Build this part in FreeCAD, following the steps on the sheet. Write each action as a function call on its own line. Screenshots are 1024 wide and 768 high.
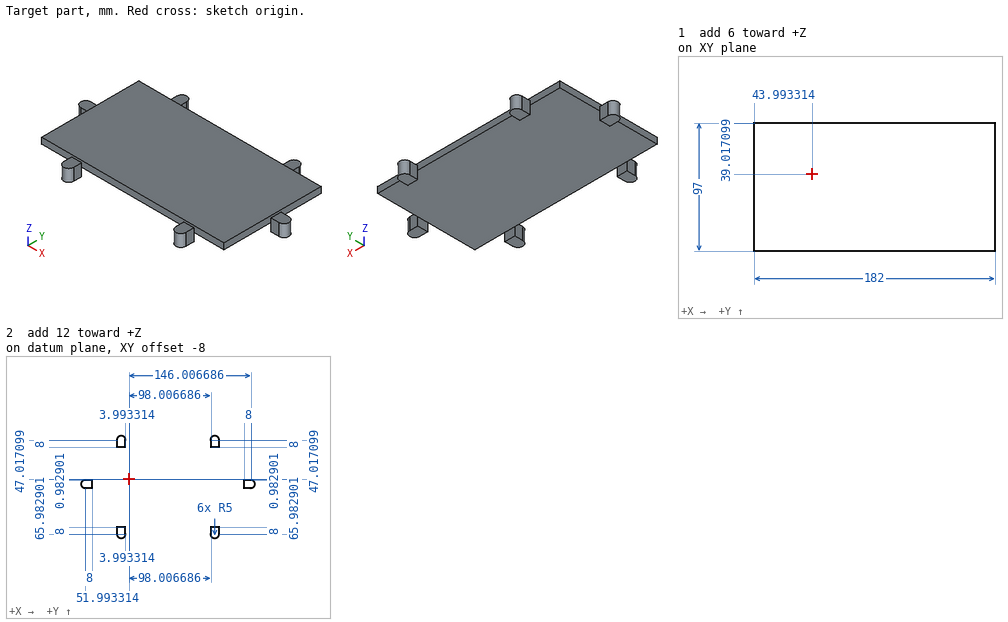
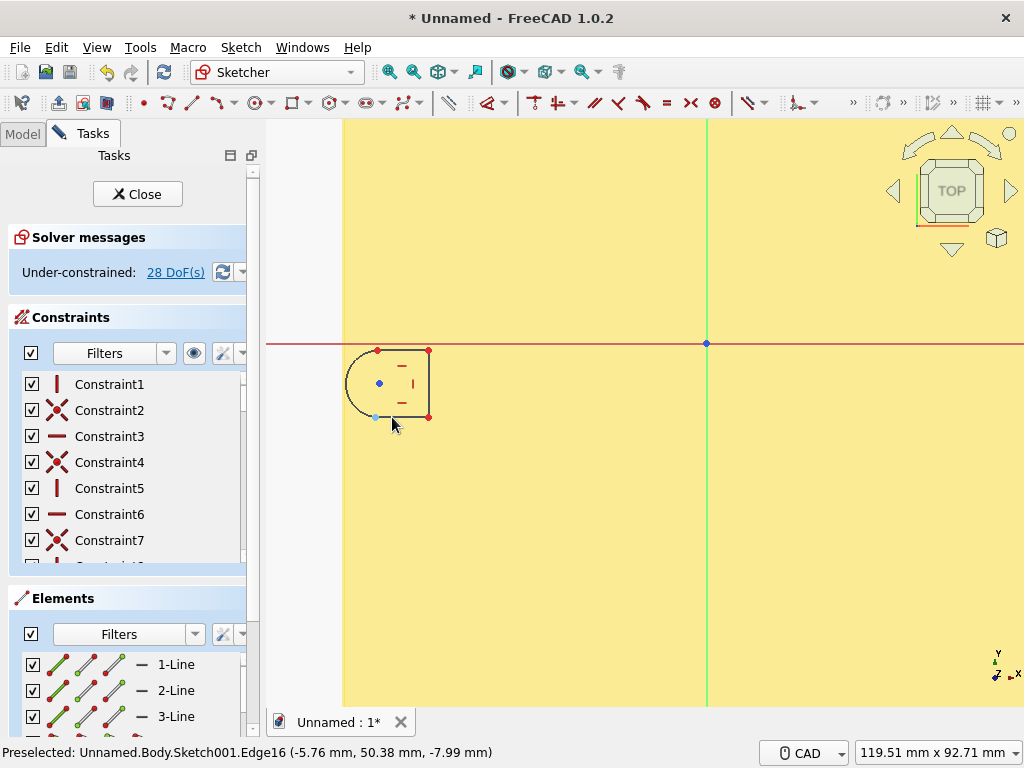
click(391, 417)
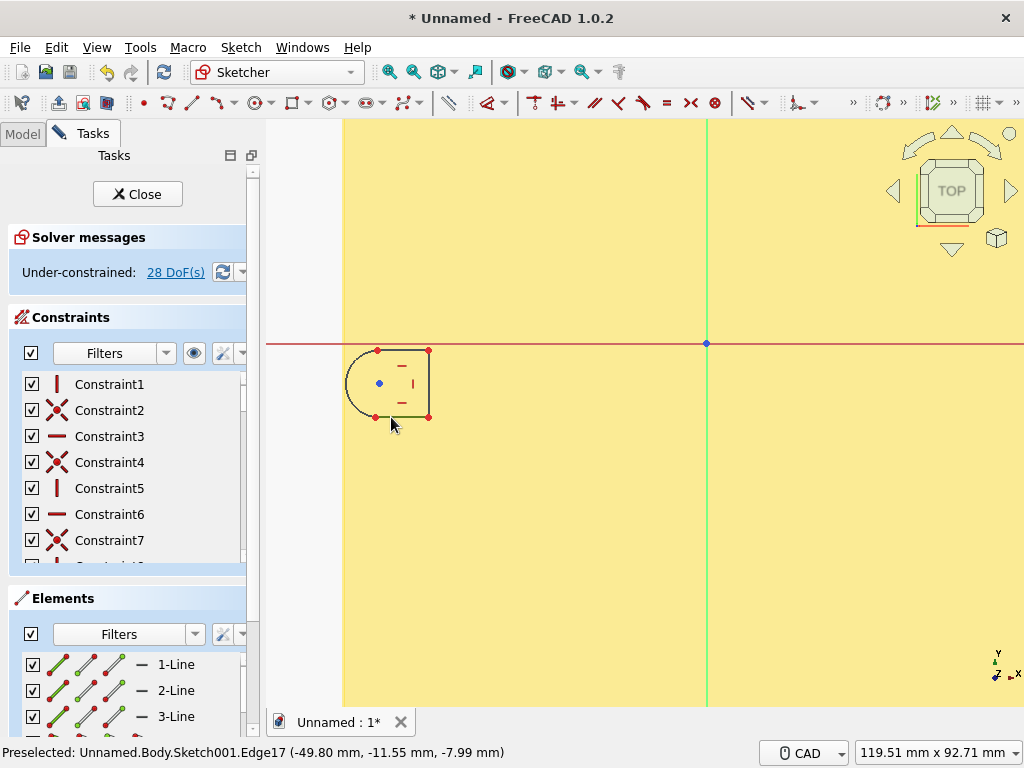
click(352, 365)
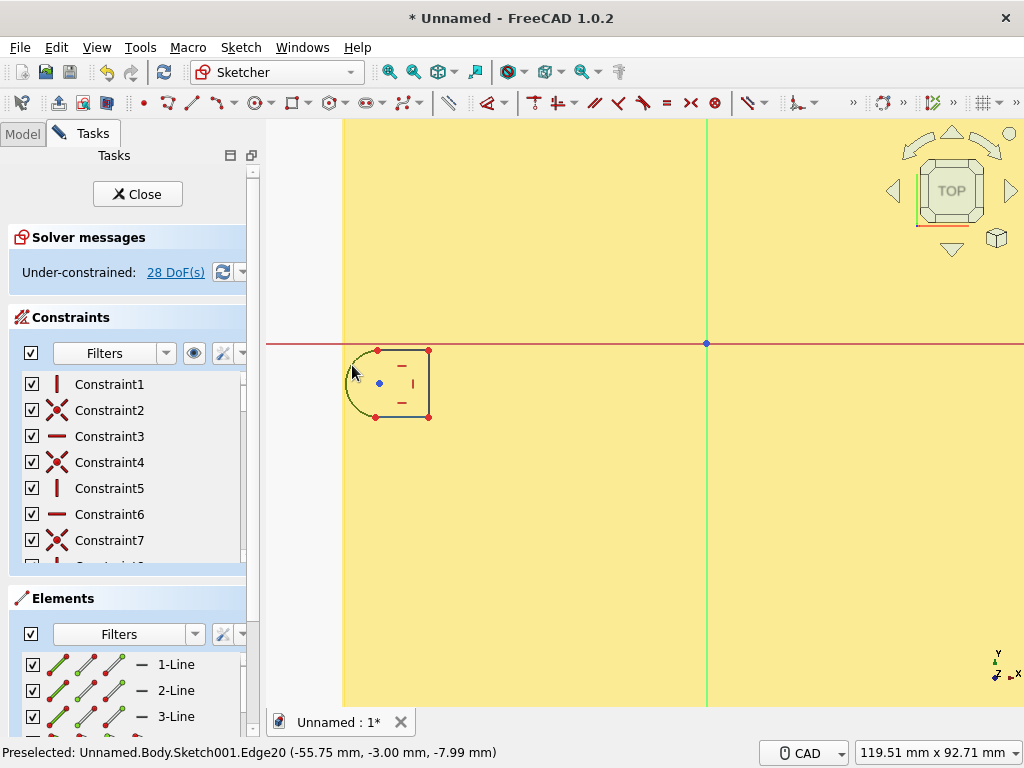
click(644, 104)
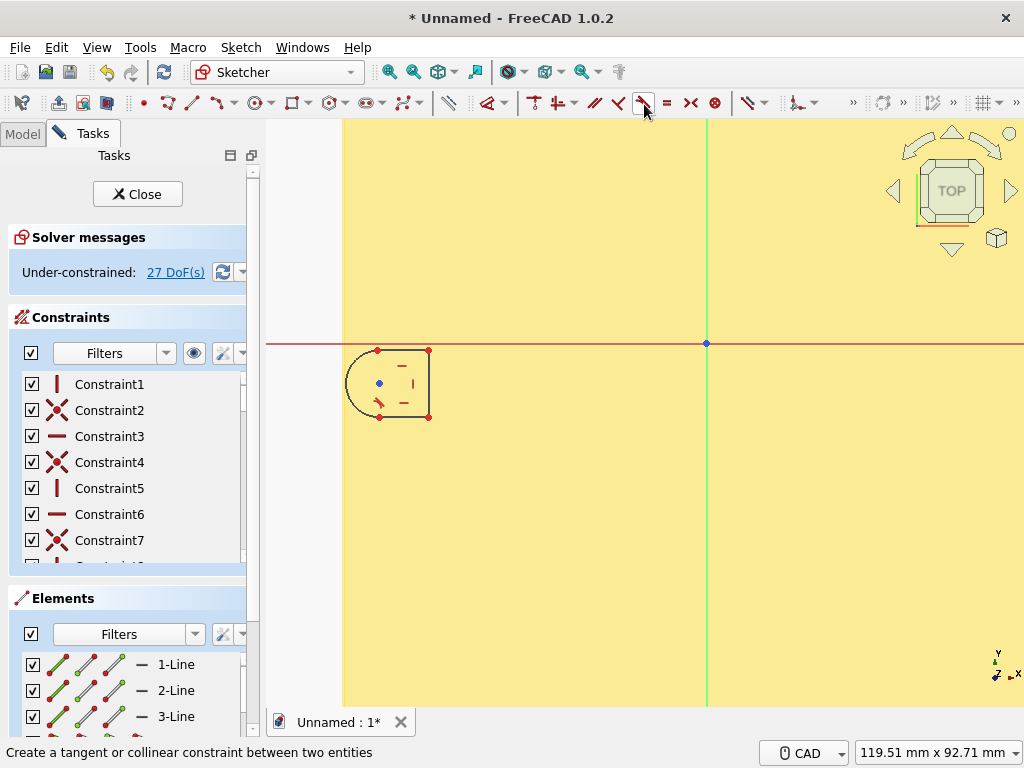
scroll(413, 350, up, 4)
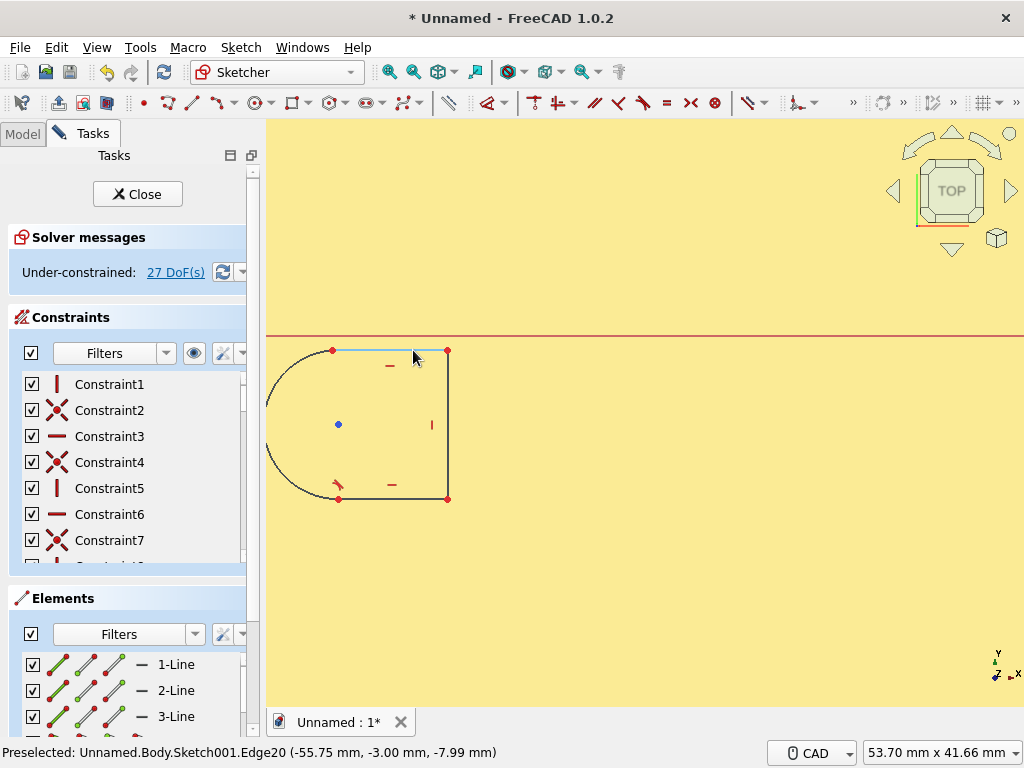
click(413, 350)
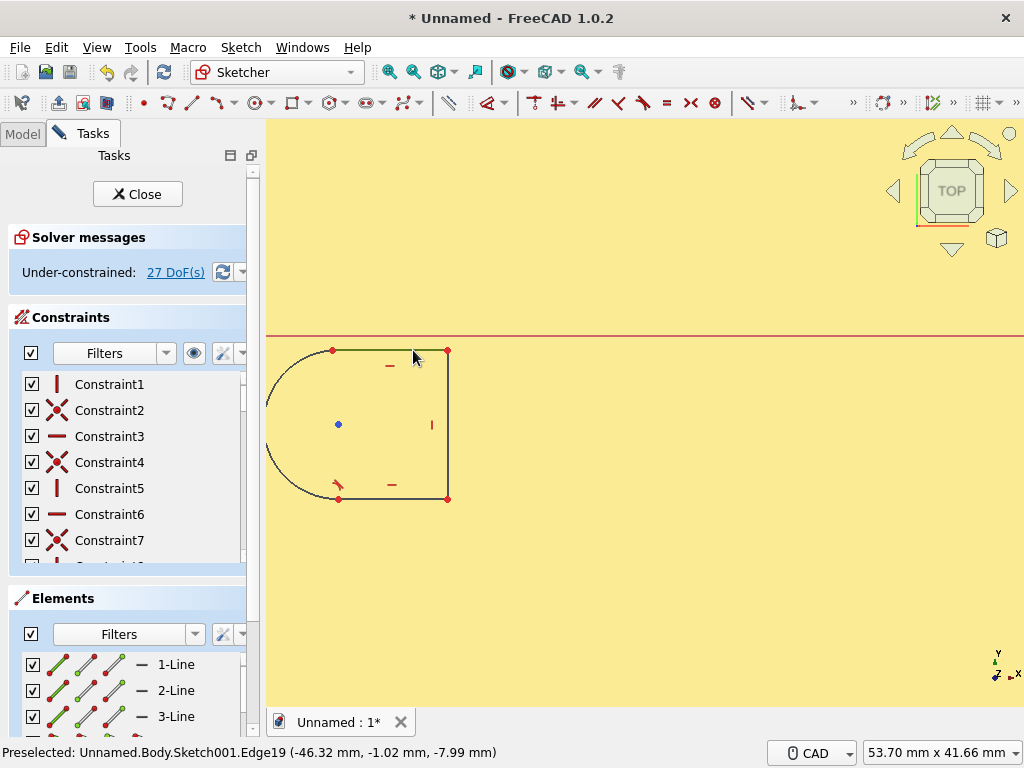
scroll(396, 404, down, 10)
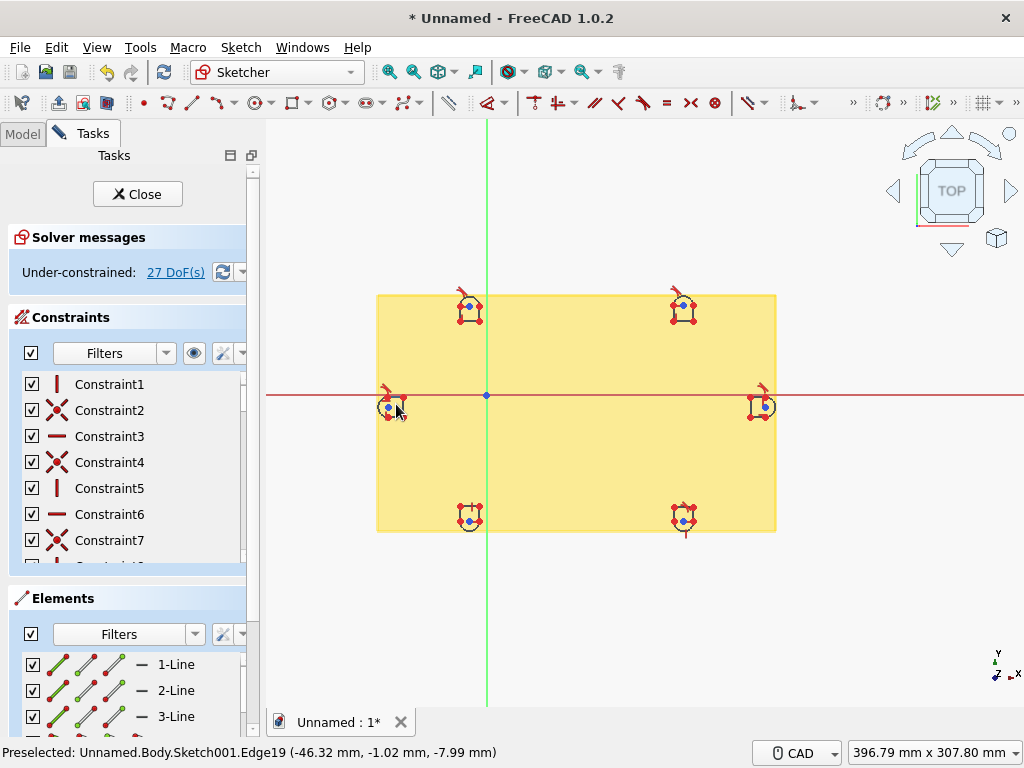
scroll(383, 415, up, 5)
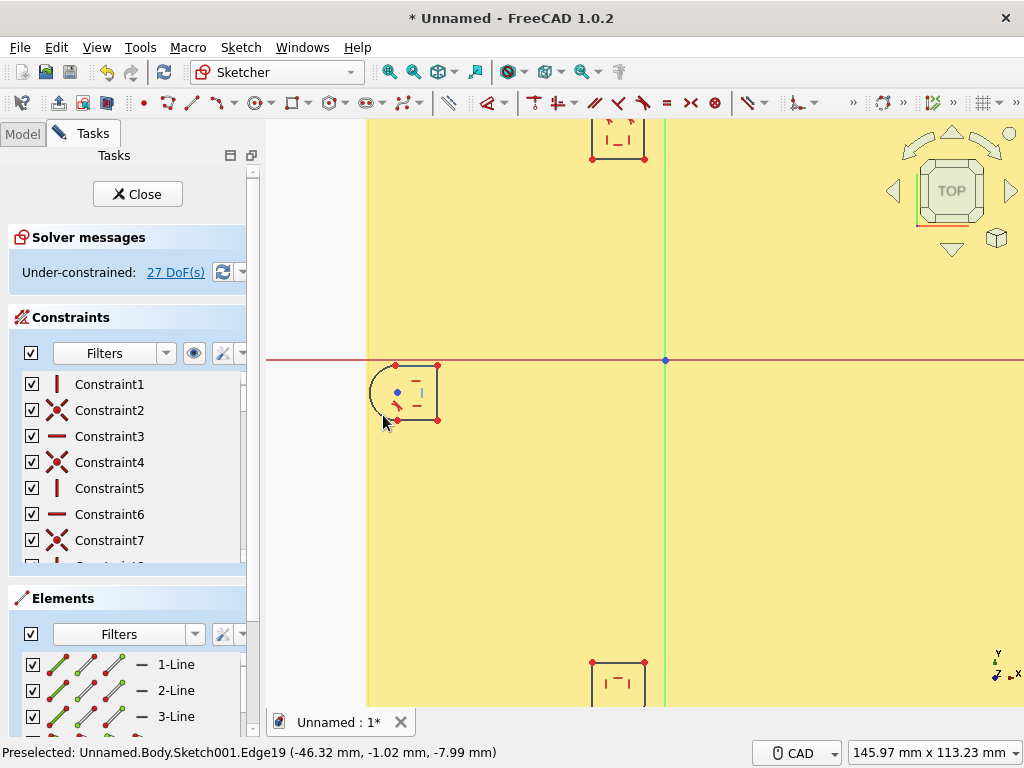
click(381, 415)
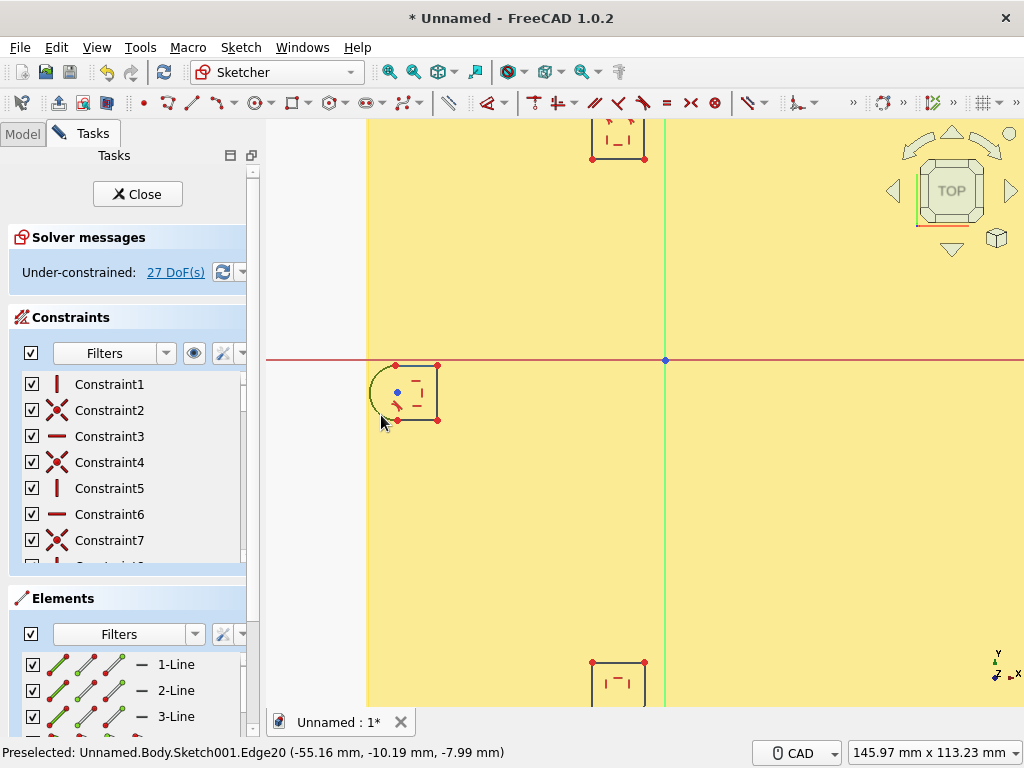
click(644, 104)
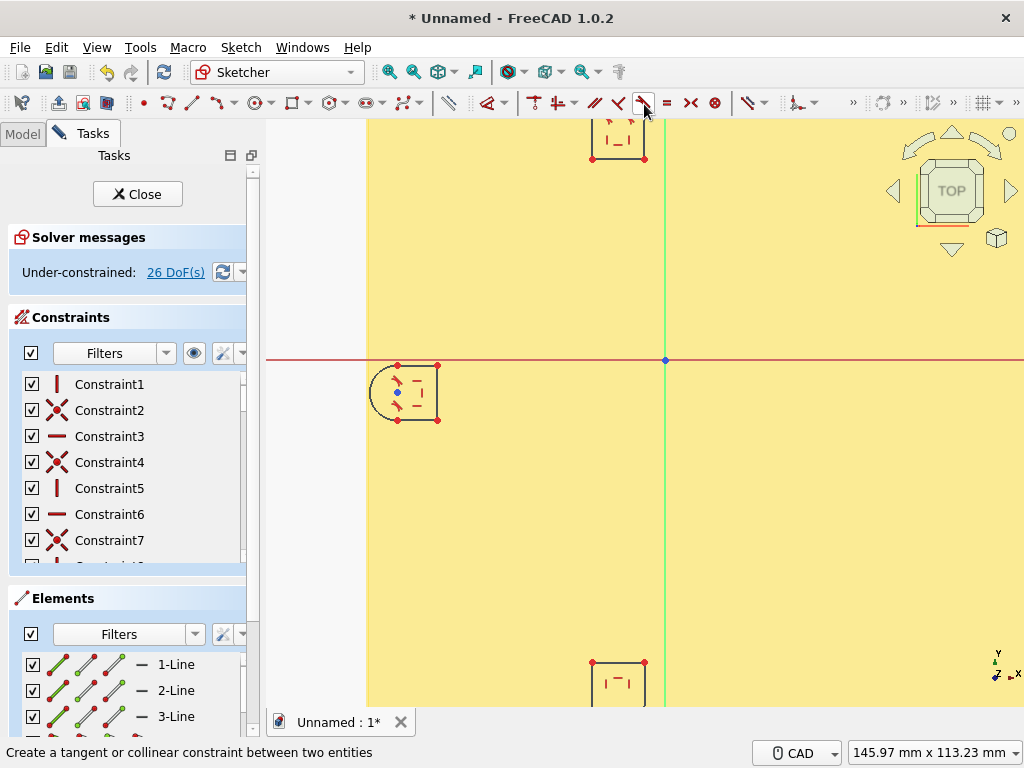
click(645, 675)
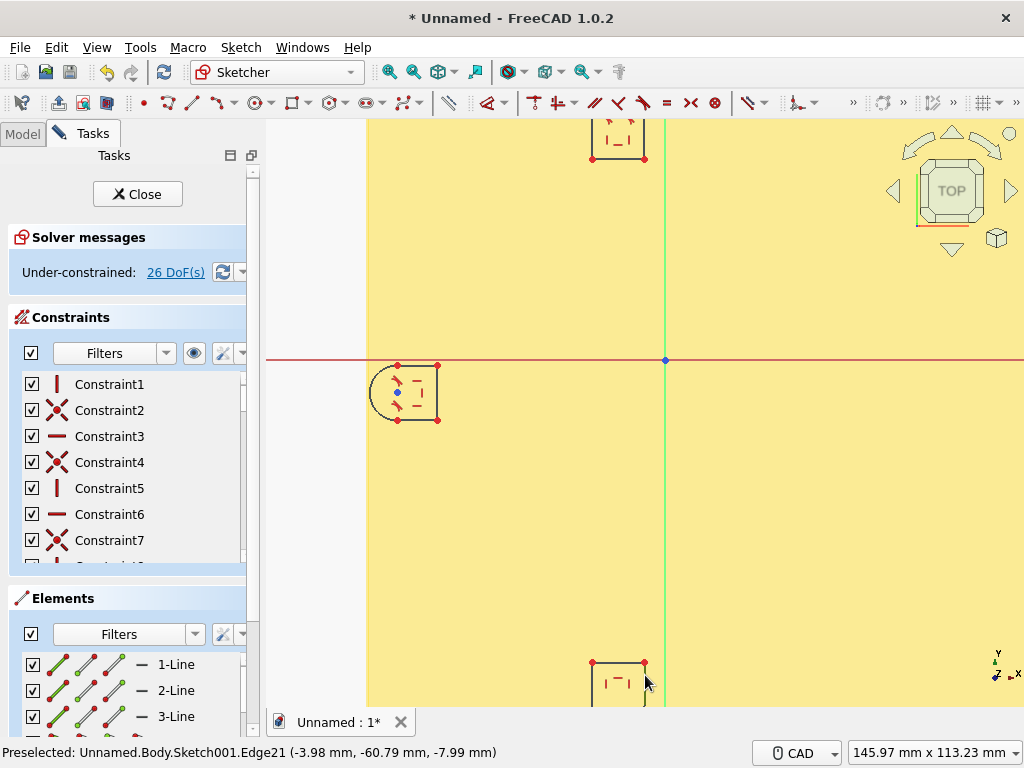
scroll(383, 415, down, 5)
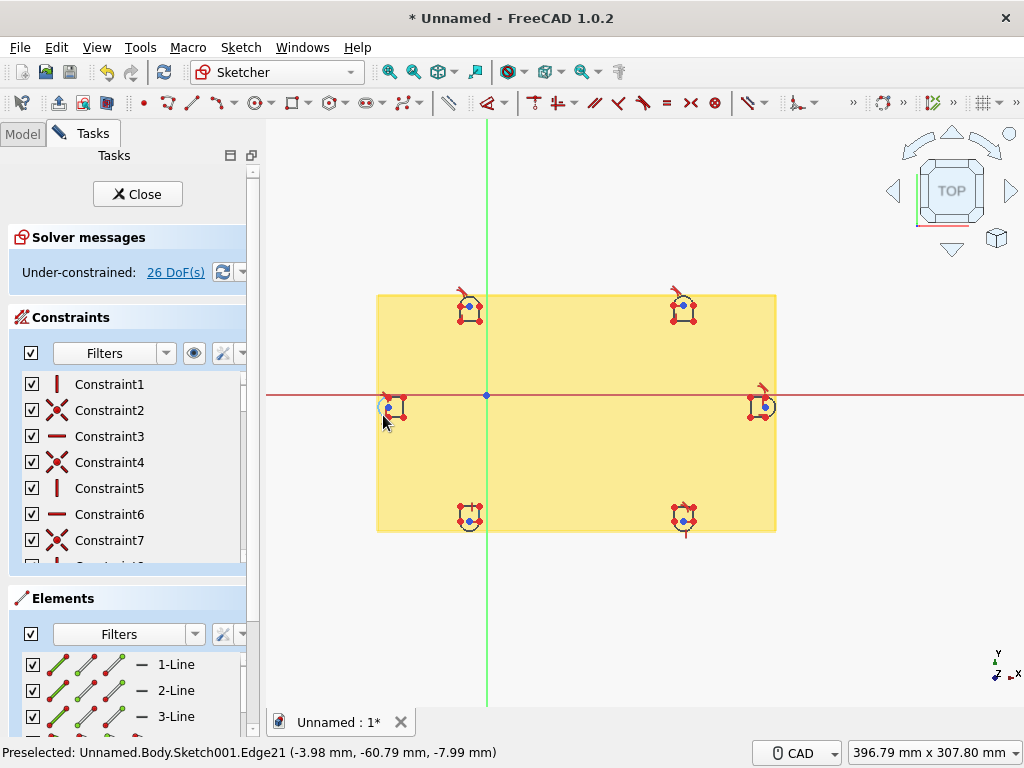
scroll(464, 529, up, 3)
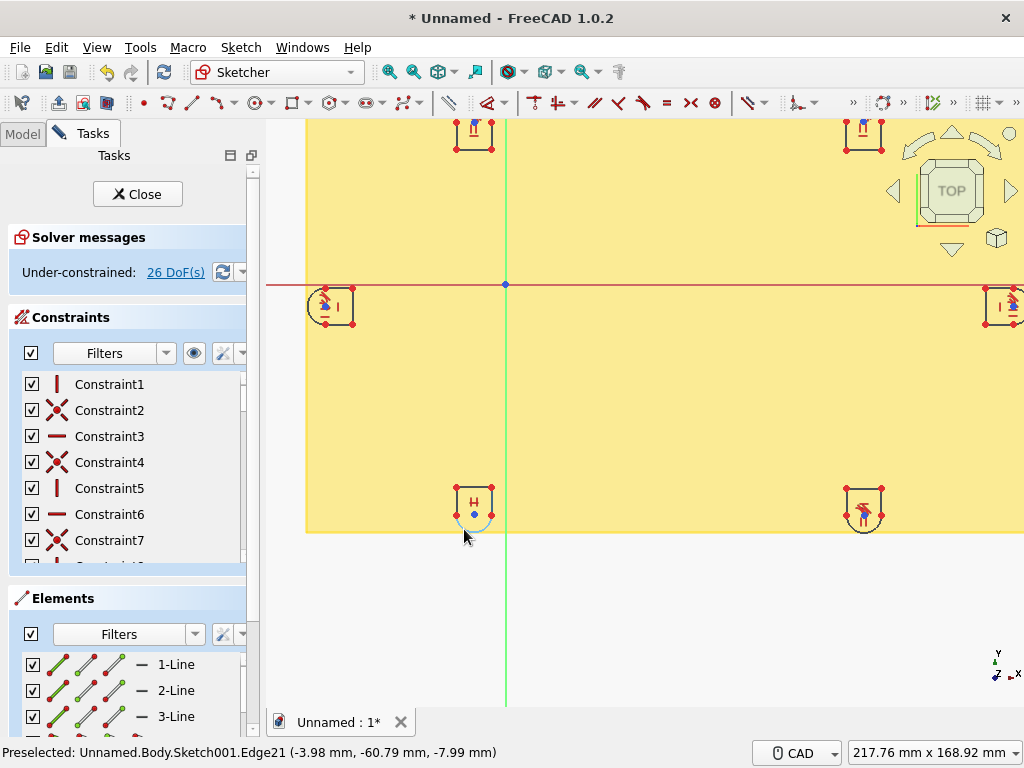
click(464, 529)